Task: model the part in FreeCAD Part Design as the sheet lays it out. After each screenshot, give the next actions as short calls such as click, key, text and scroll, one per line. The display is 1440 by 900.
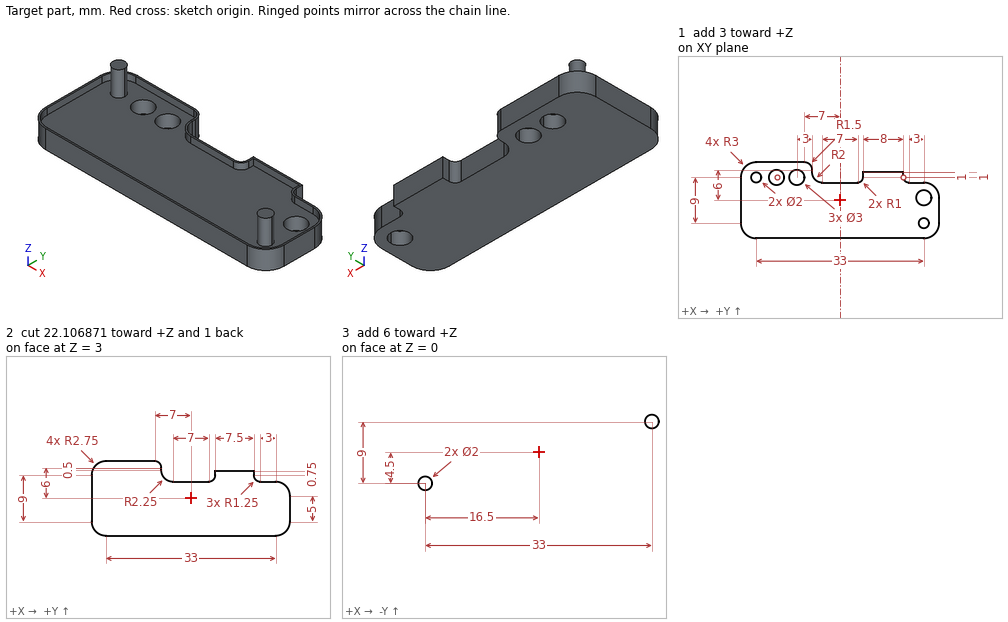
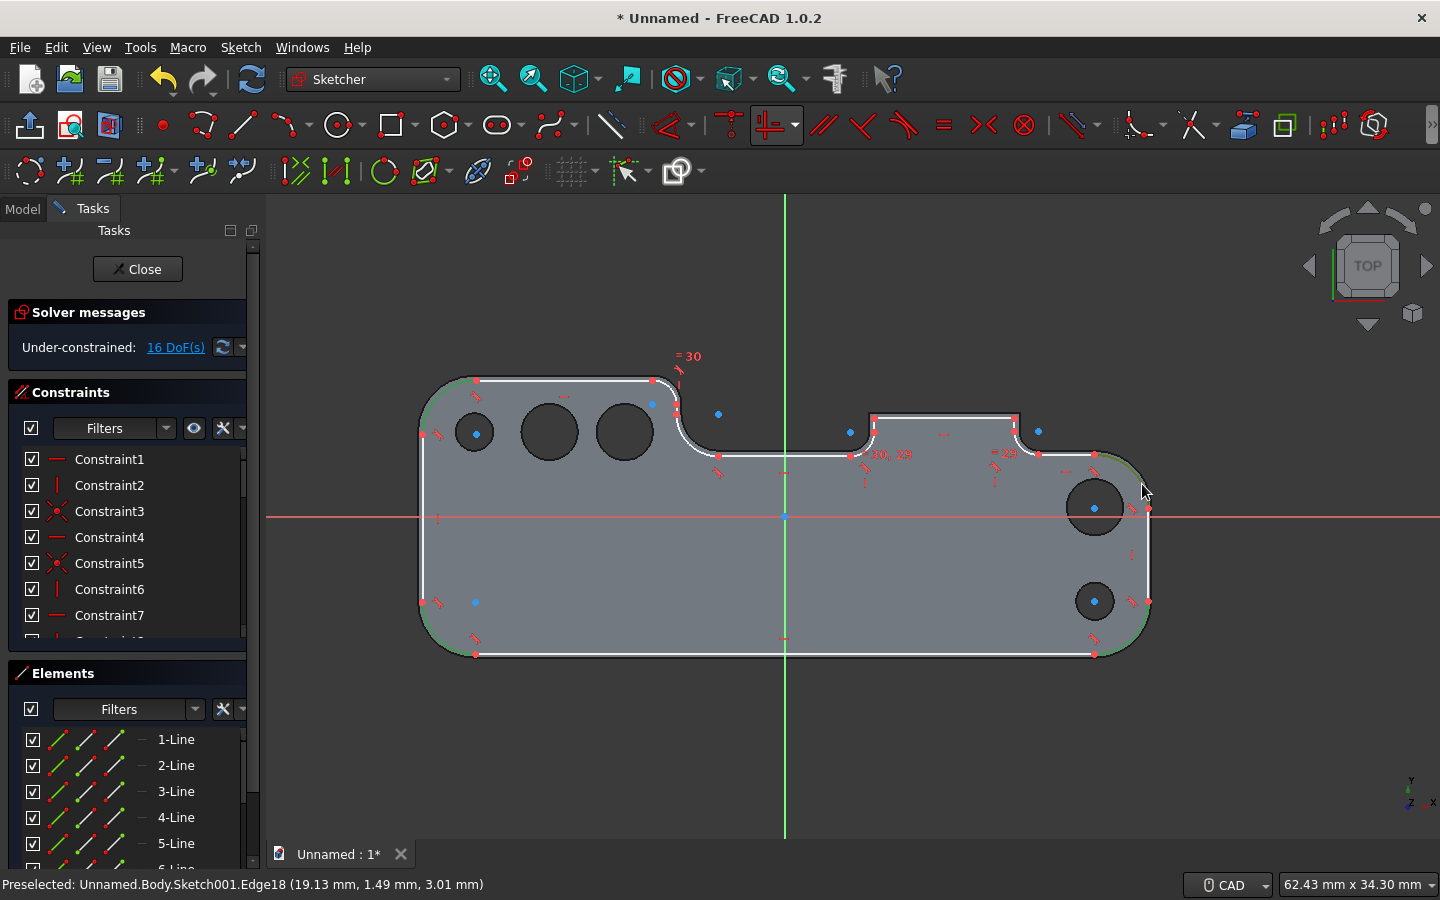
click(944, 126)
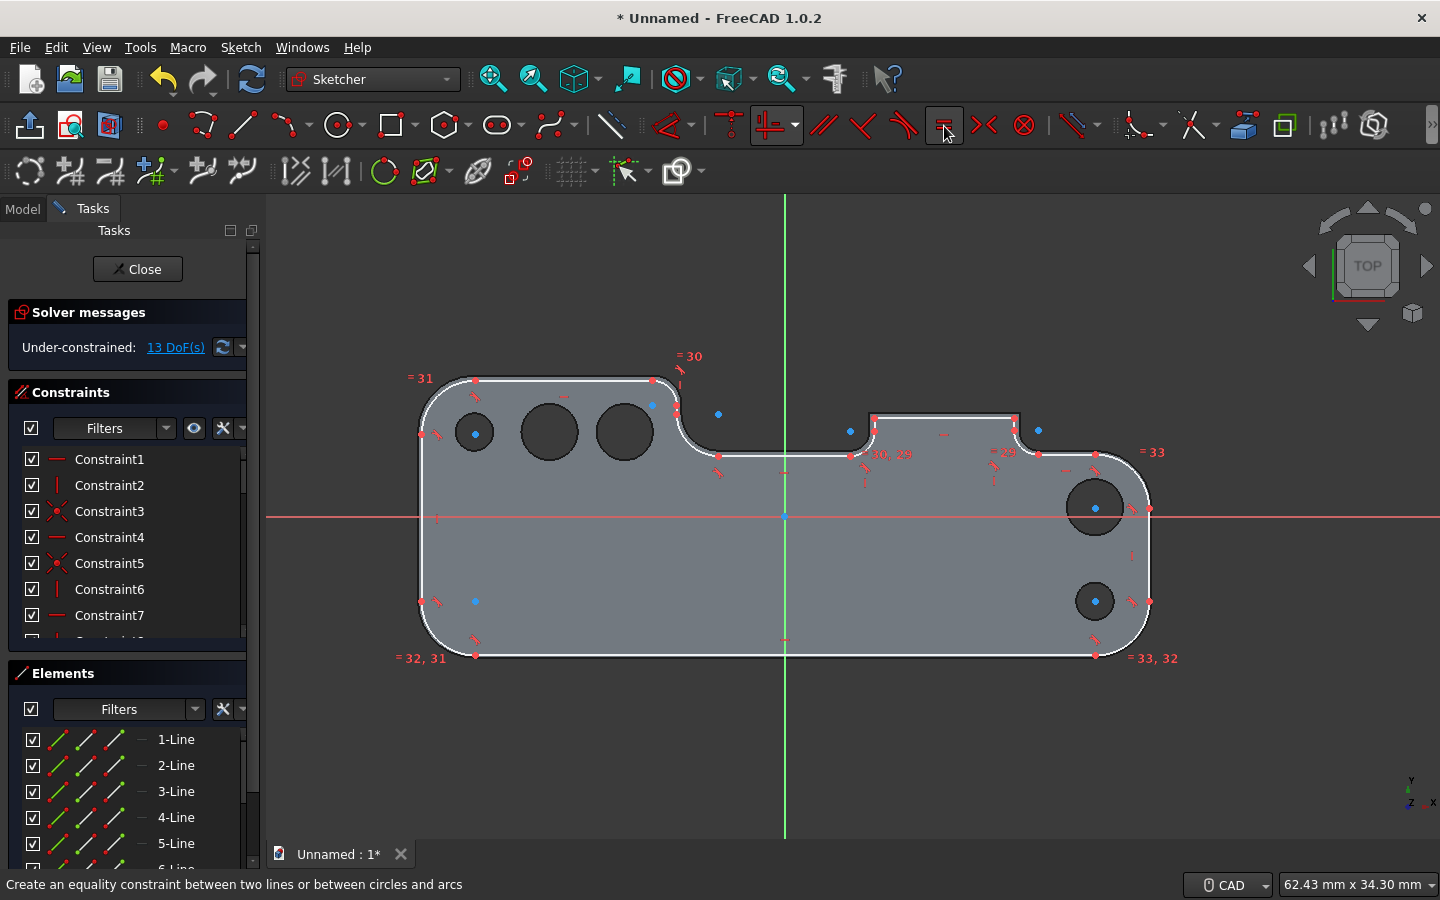
click(666, 126)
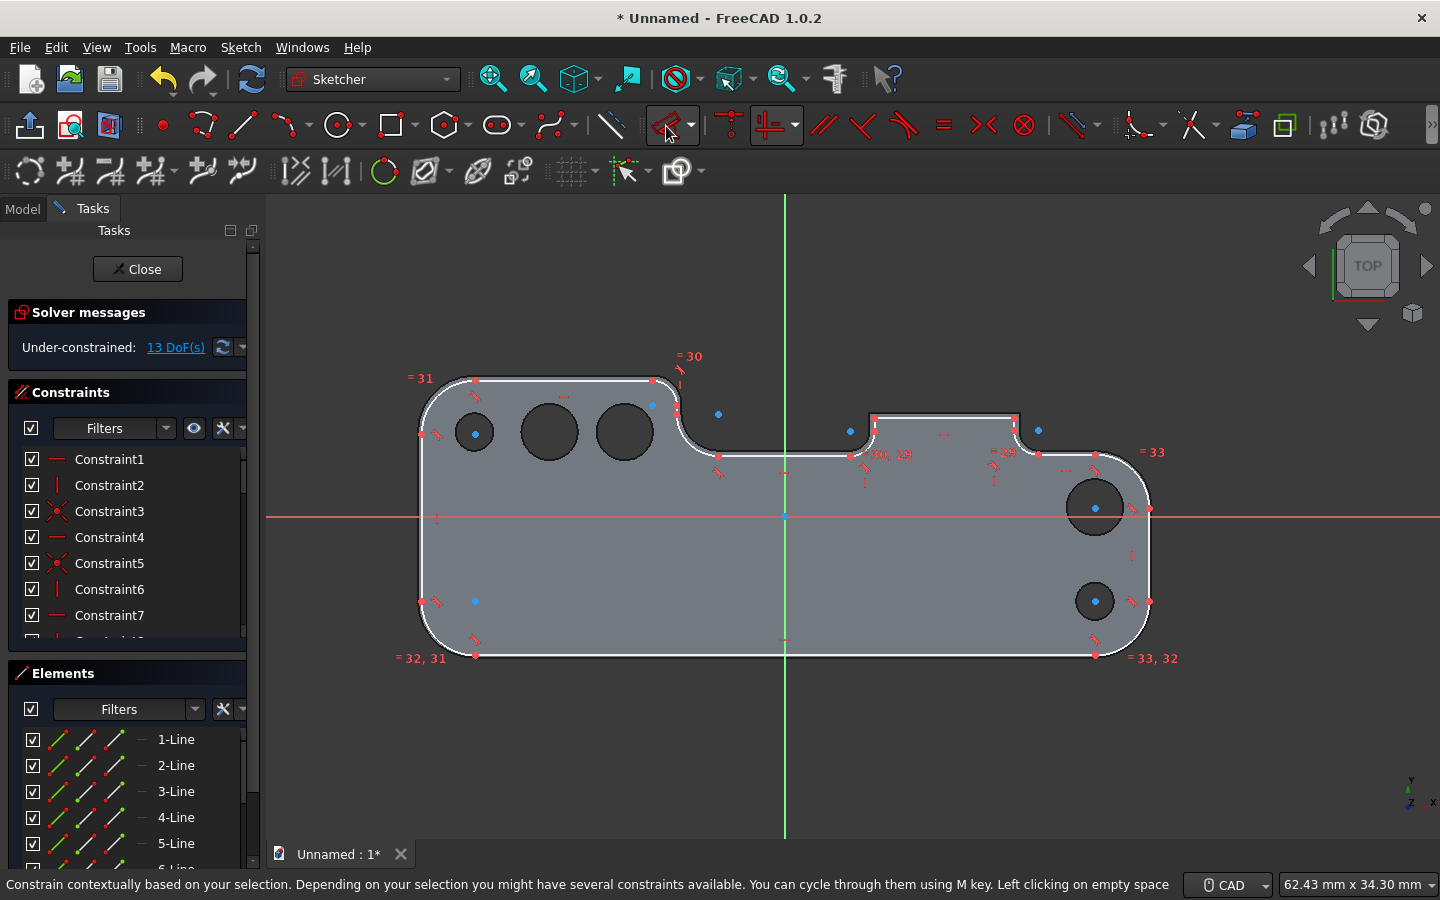
scroll(1017, 442, up, 3)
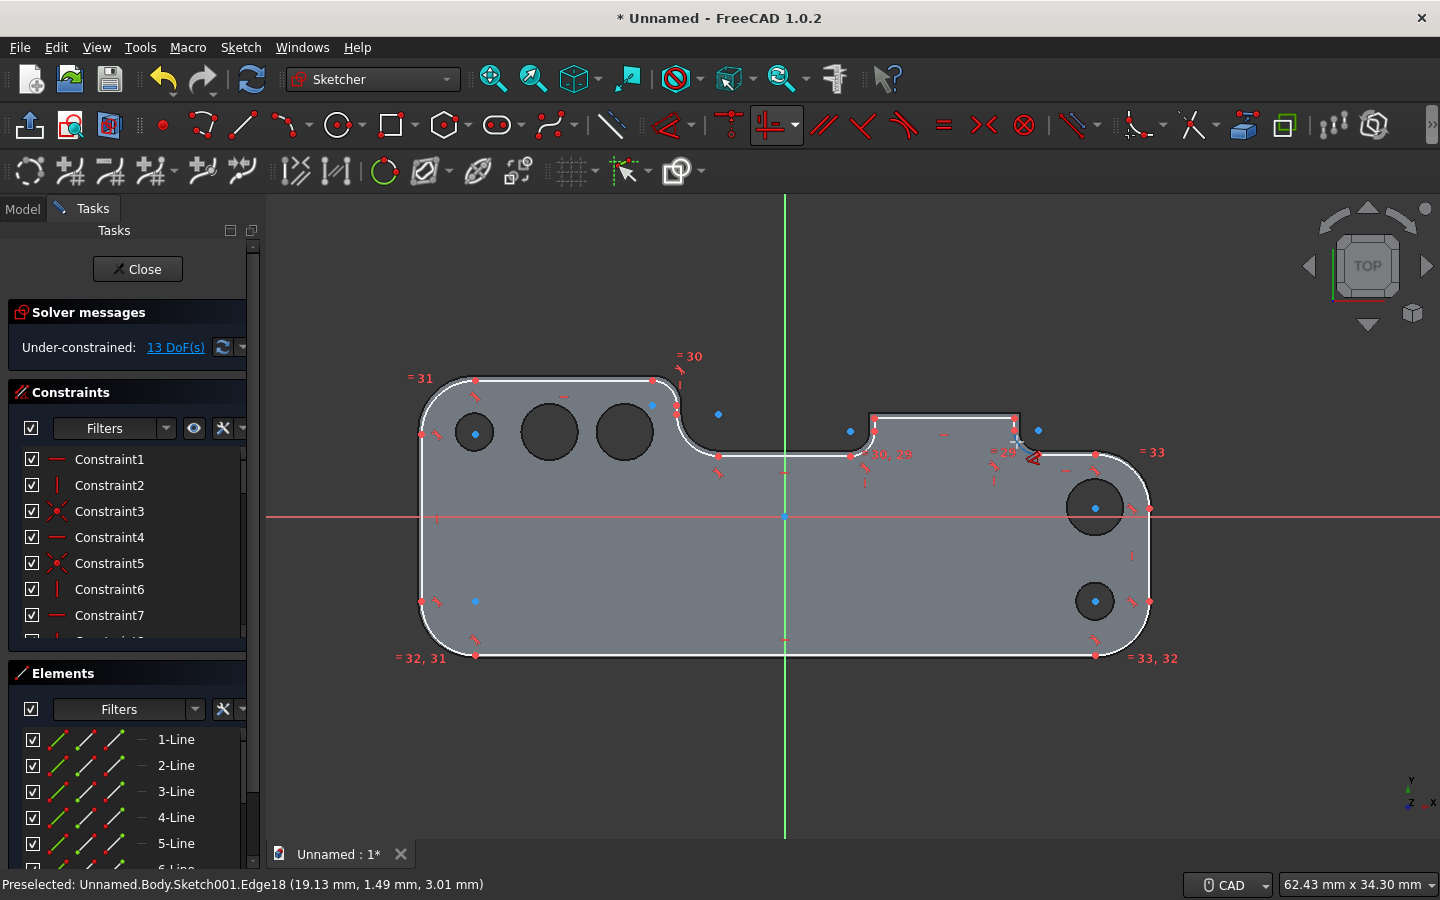
click(1016, 441)
click(988, 456)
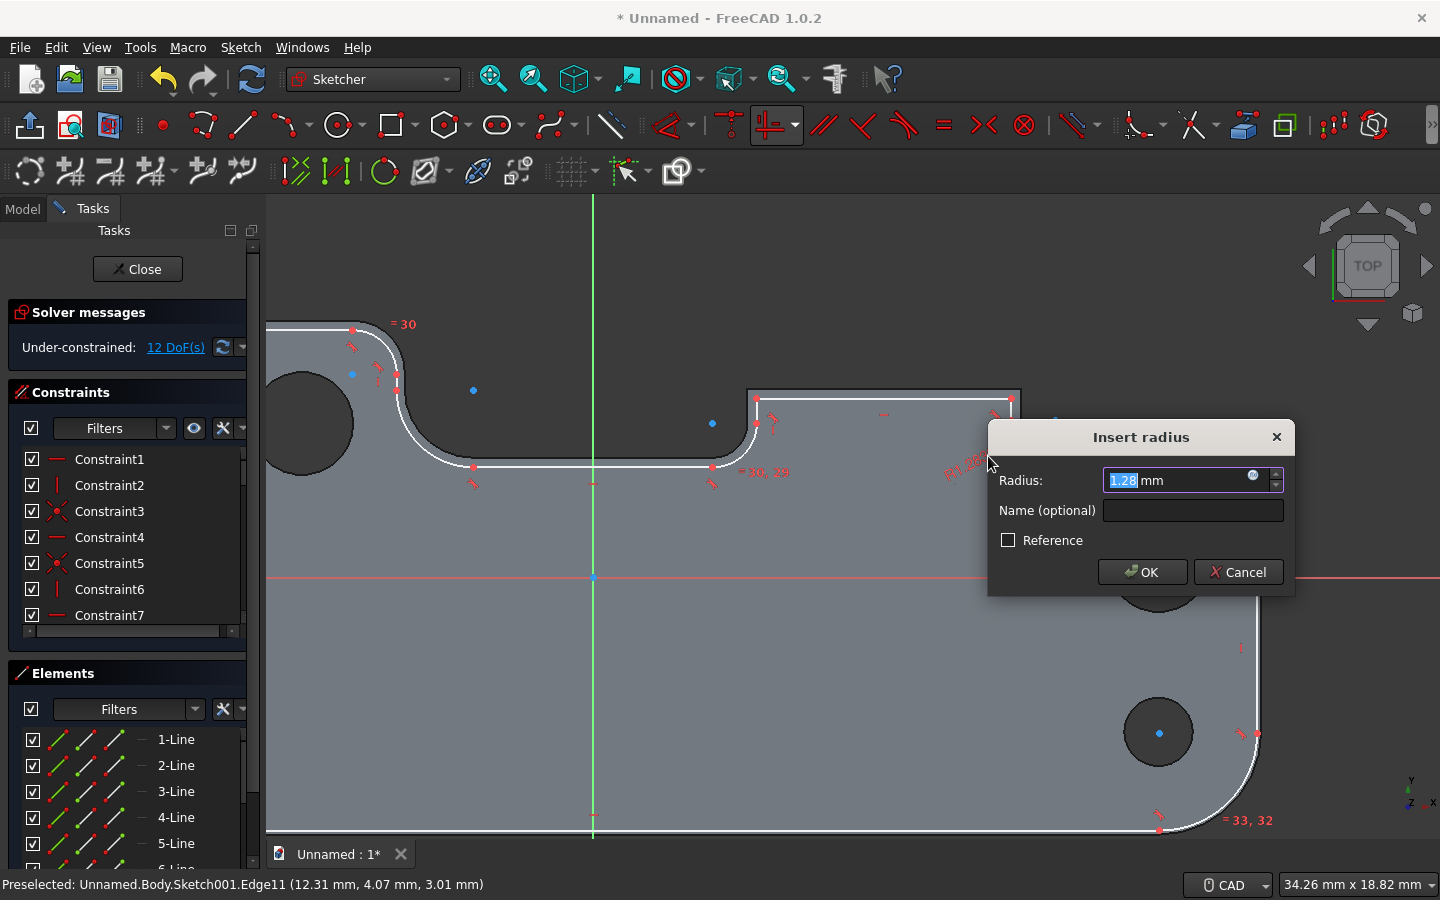
text(1.25)
key(Return)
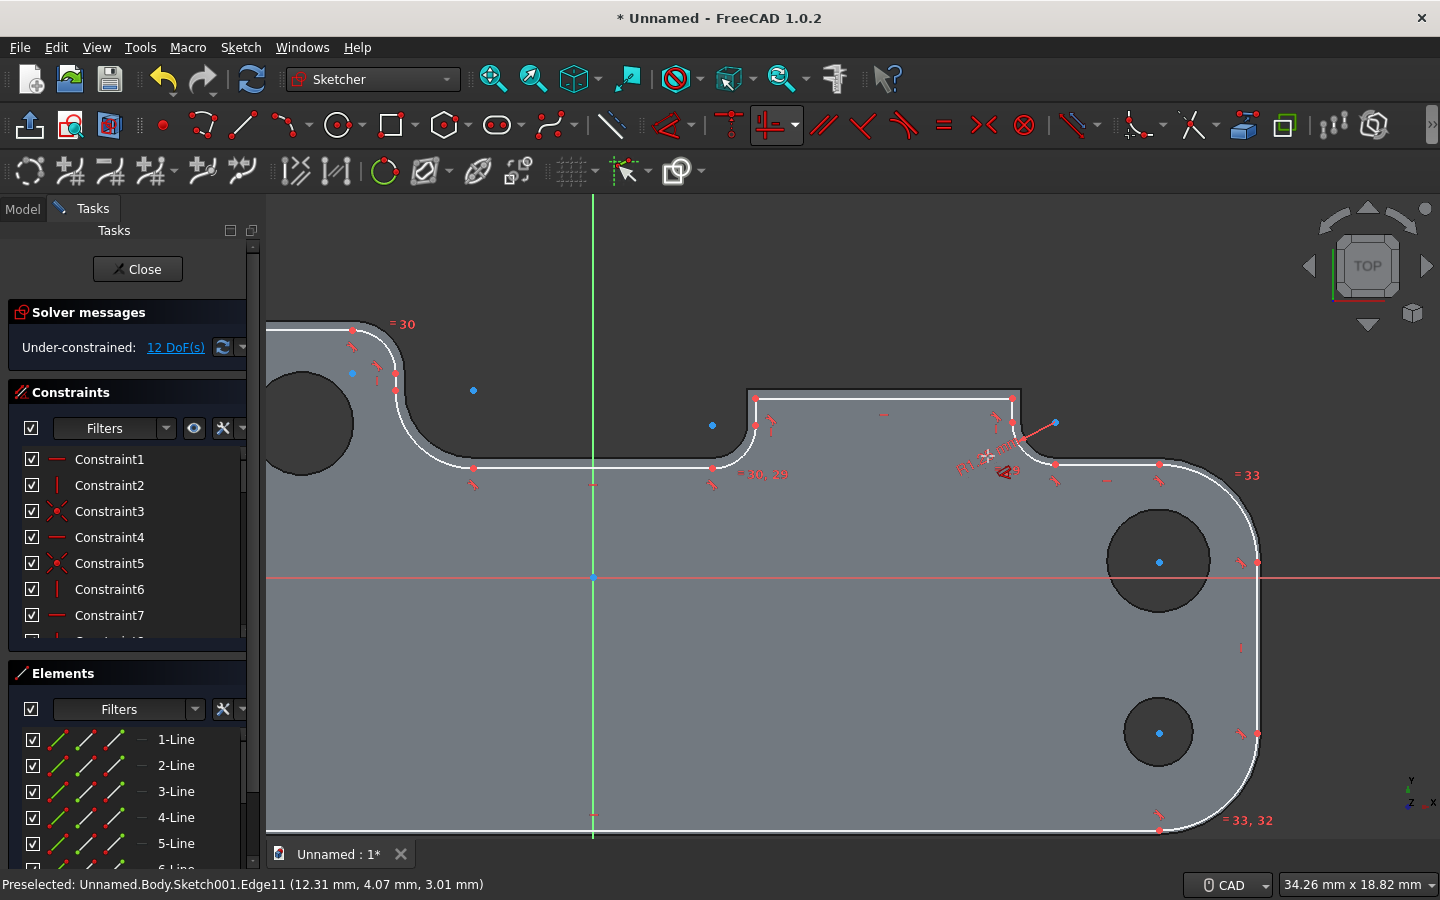
click(404, 426)
click(375, 441)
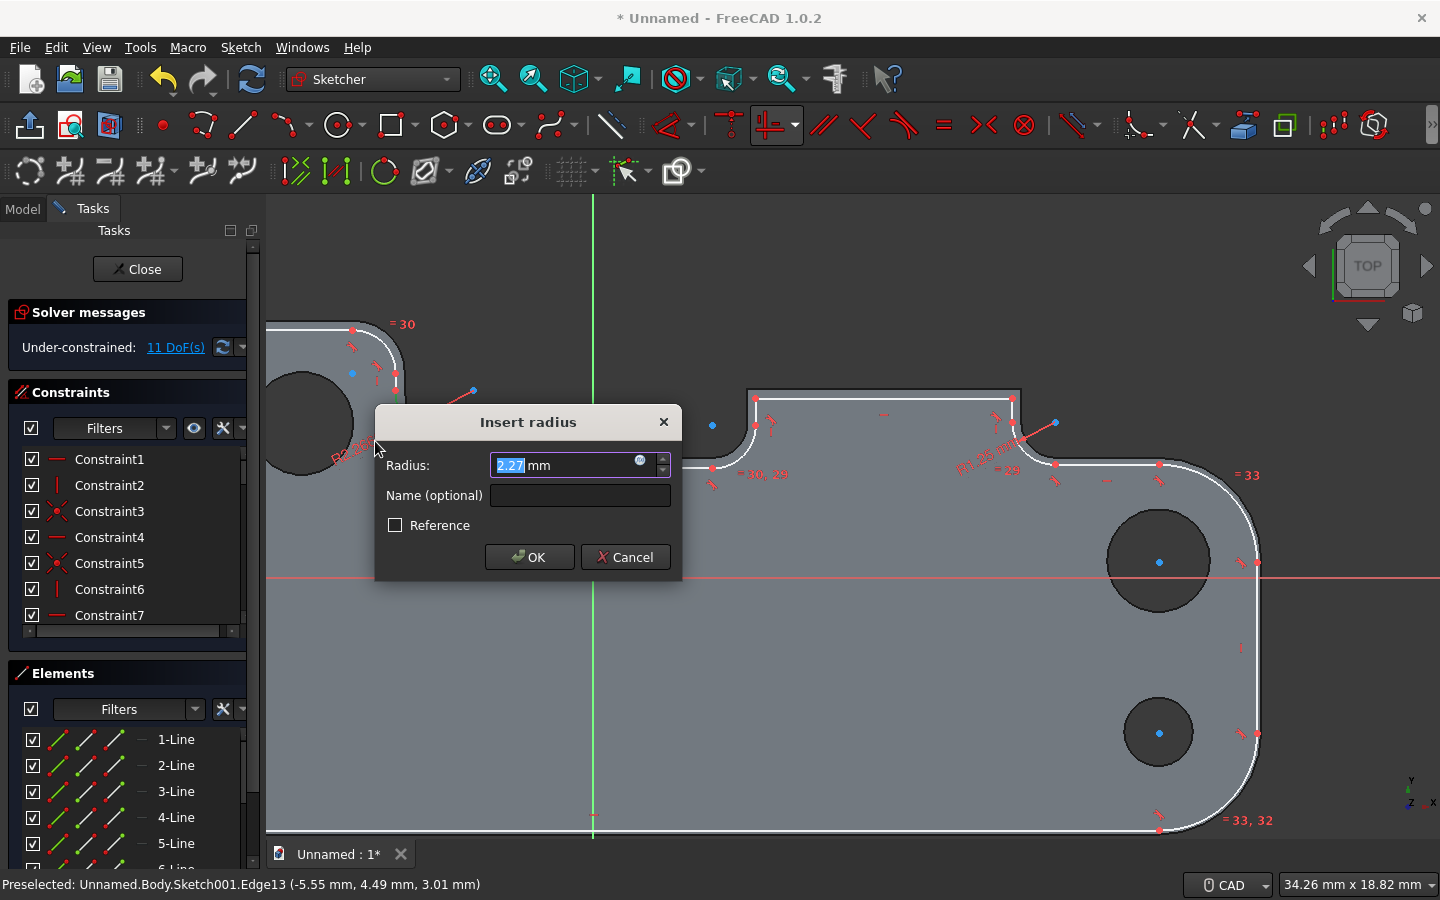
text(2.25)
key(Return)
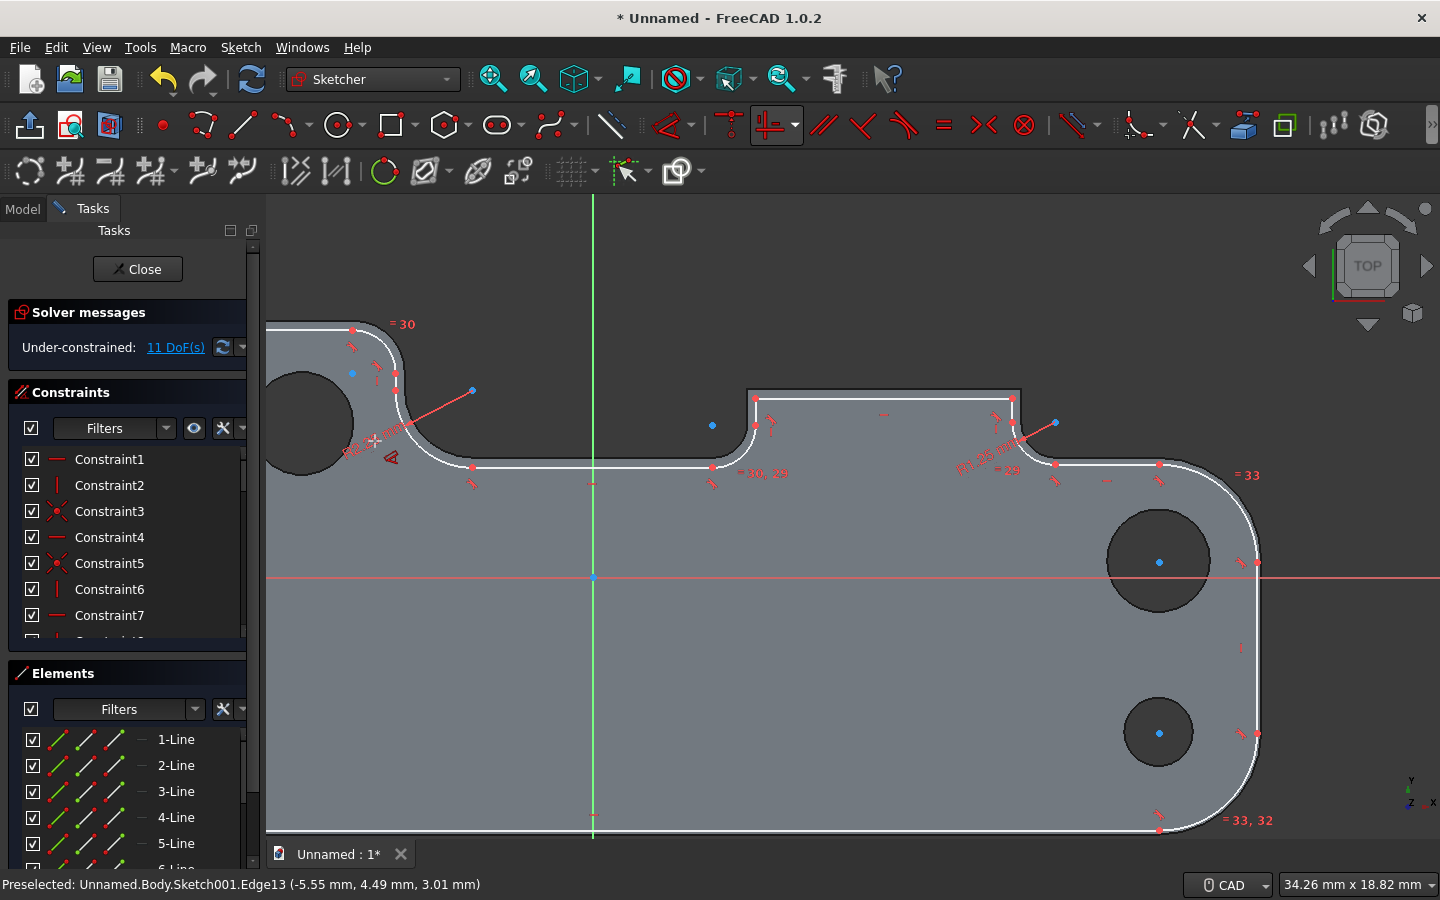
scroll(1017, 442, down, 3)